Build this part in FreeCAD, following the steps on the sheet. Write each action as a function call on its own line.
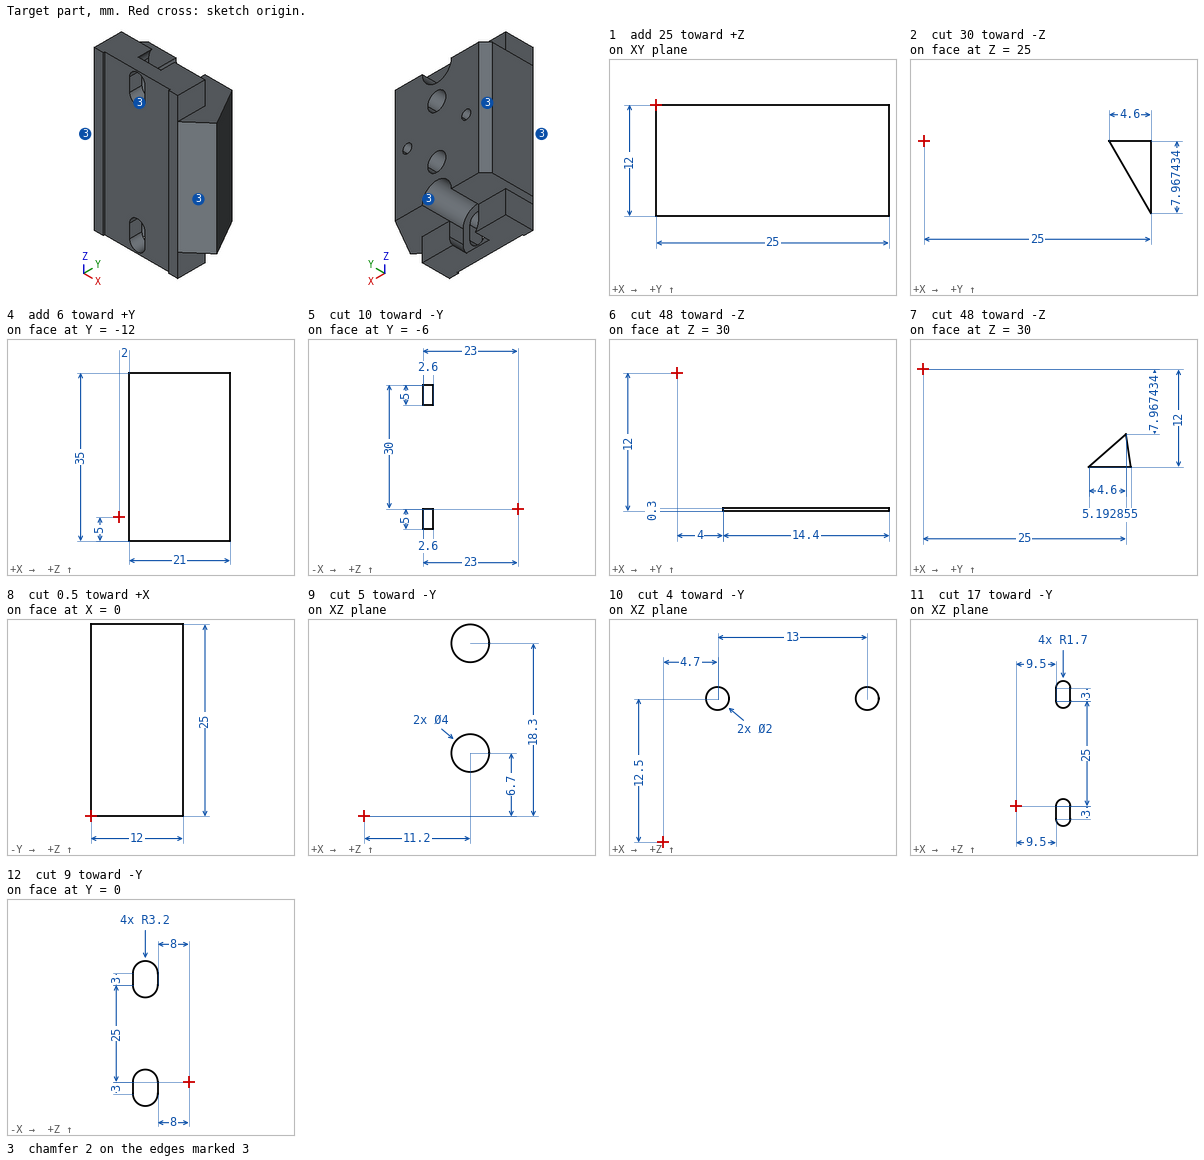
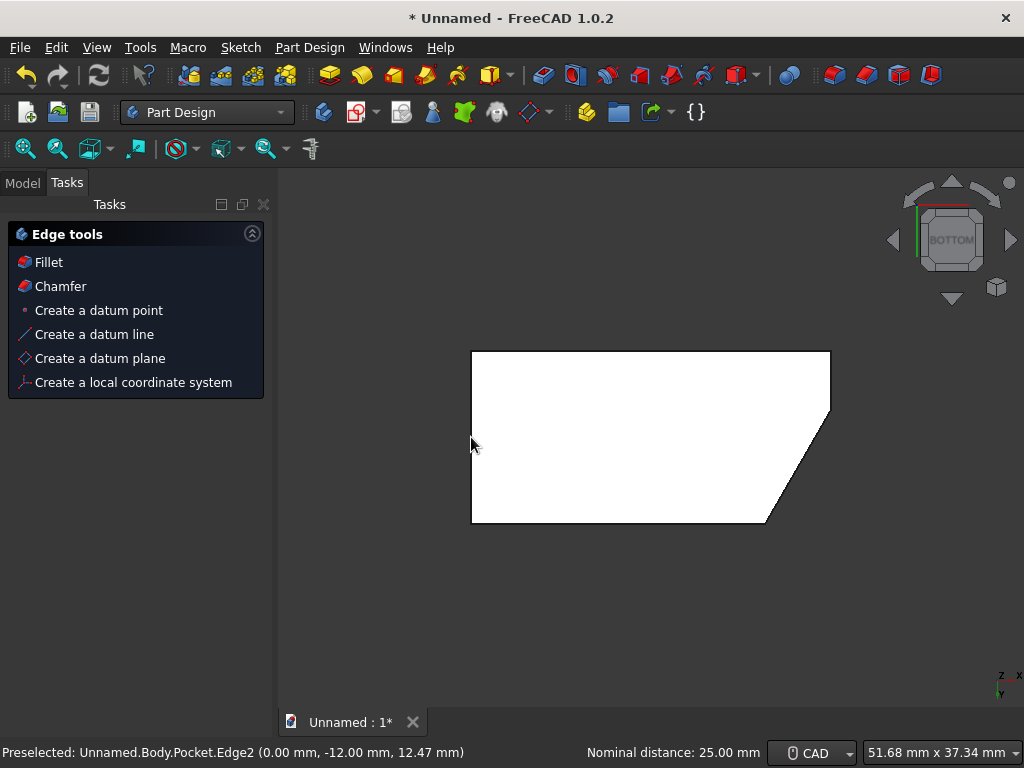
key(4)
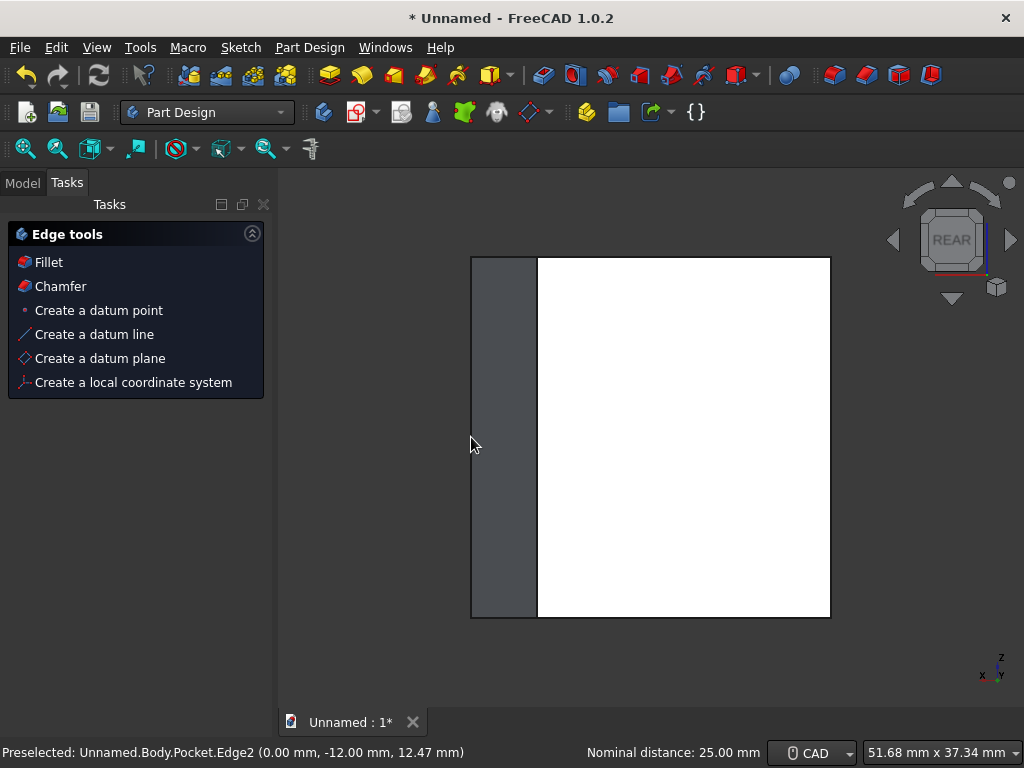
click(831, 437, ctrl)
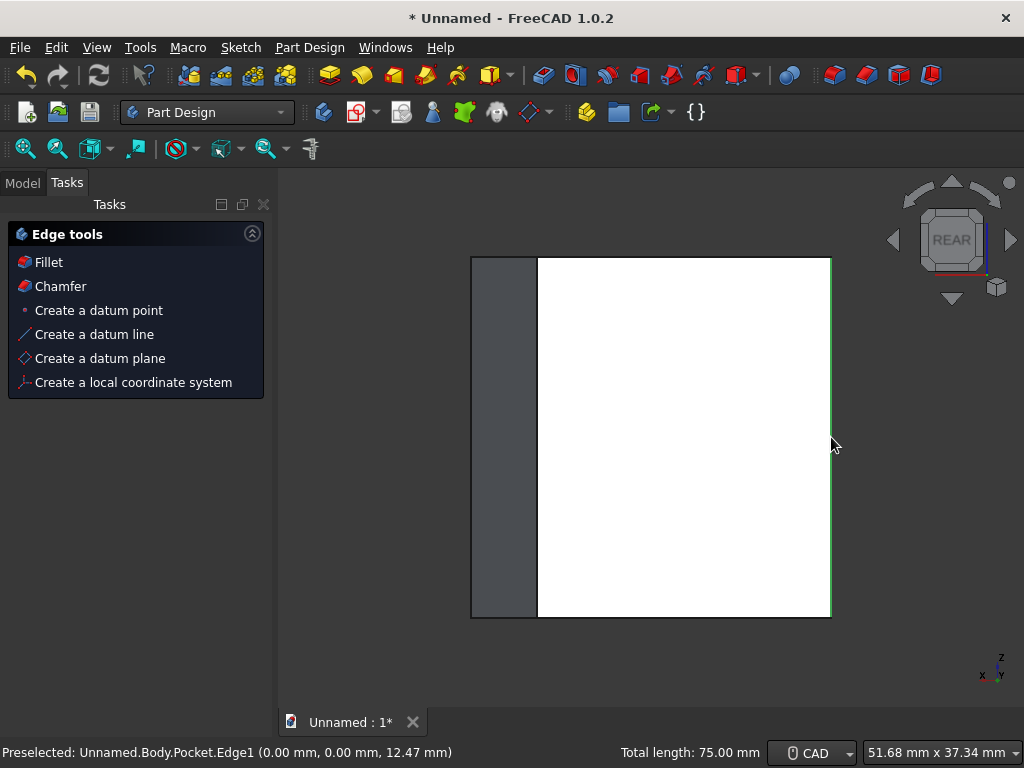
click(868, 76)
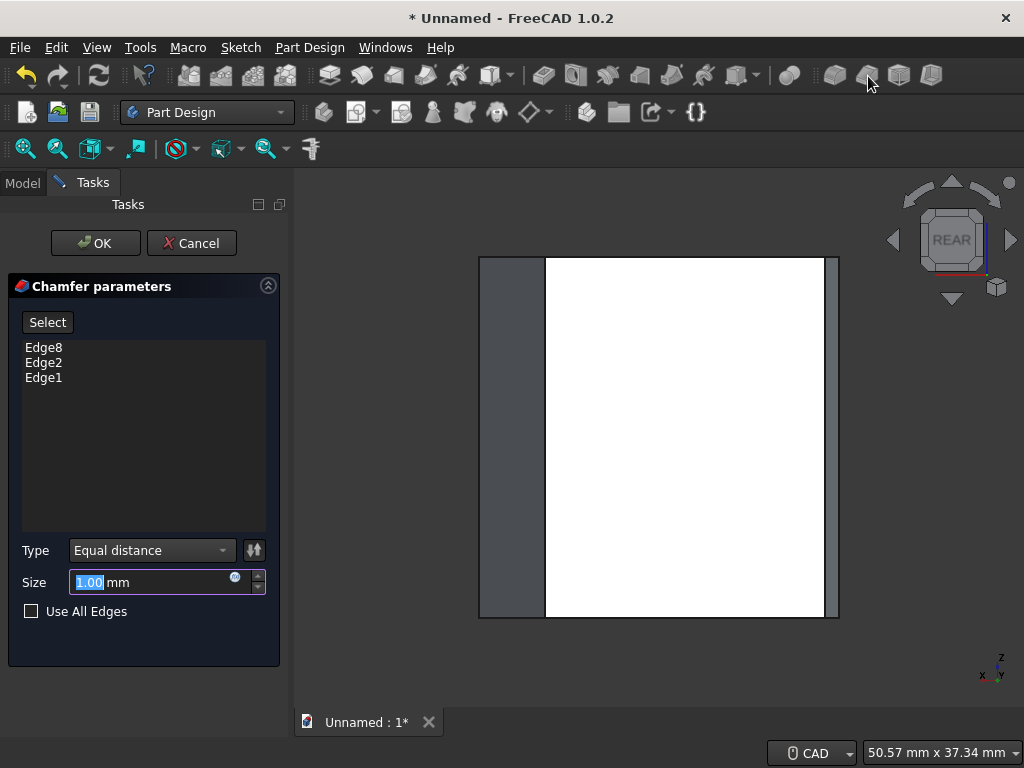
text(2)
key(Tab)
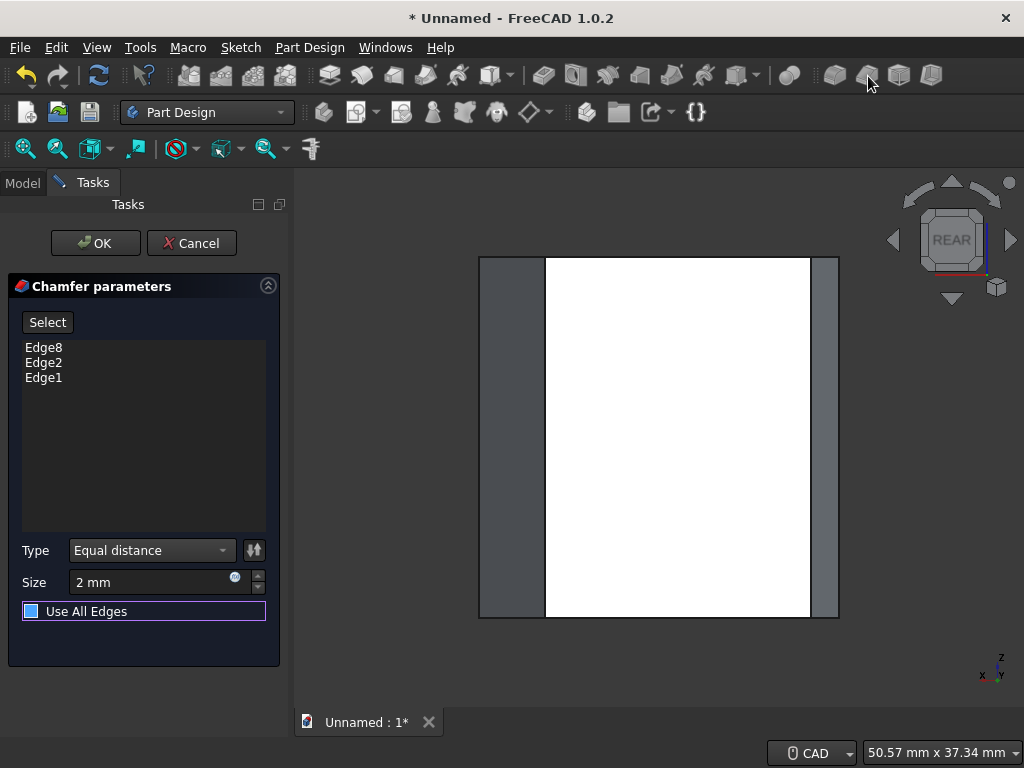
click(96, 243)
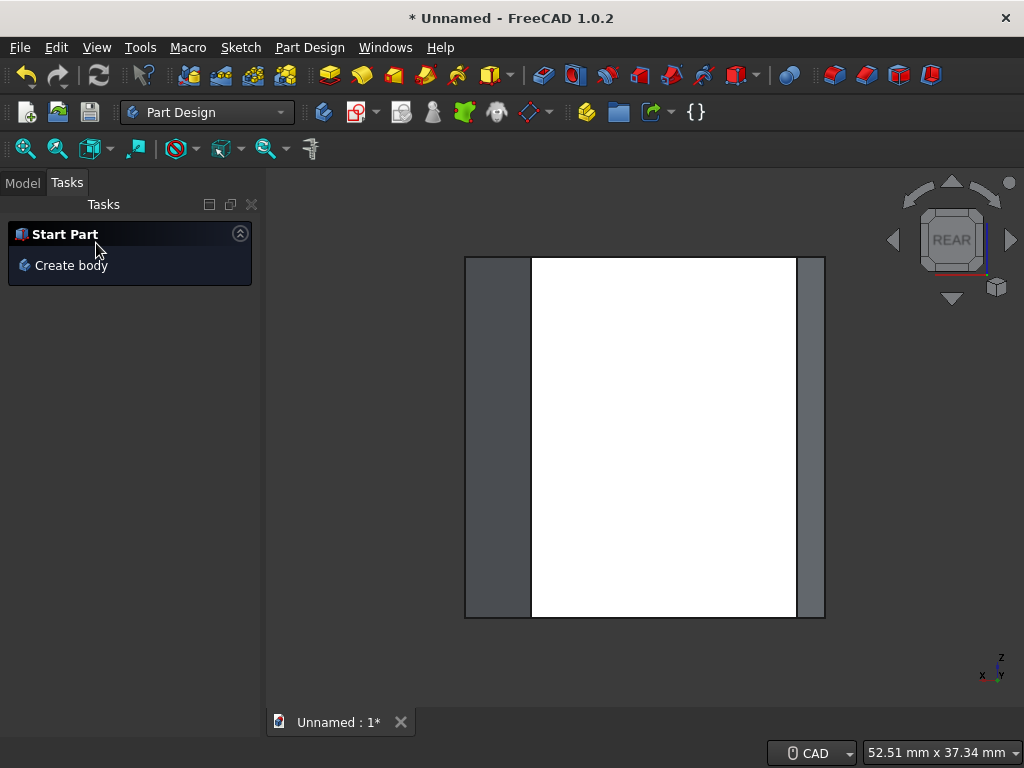
key(0)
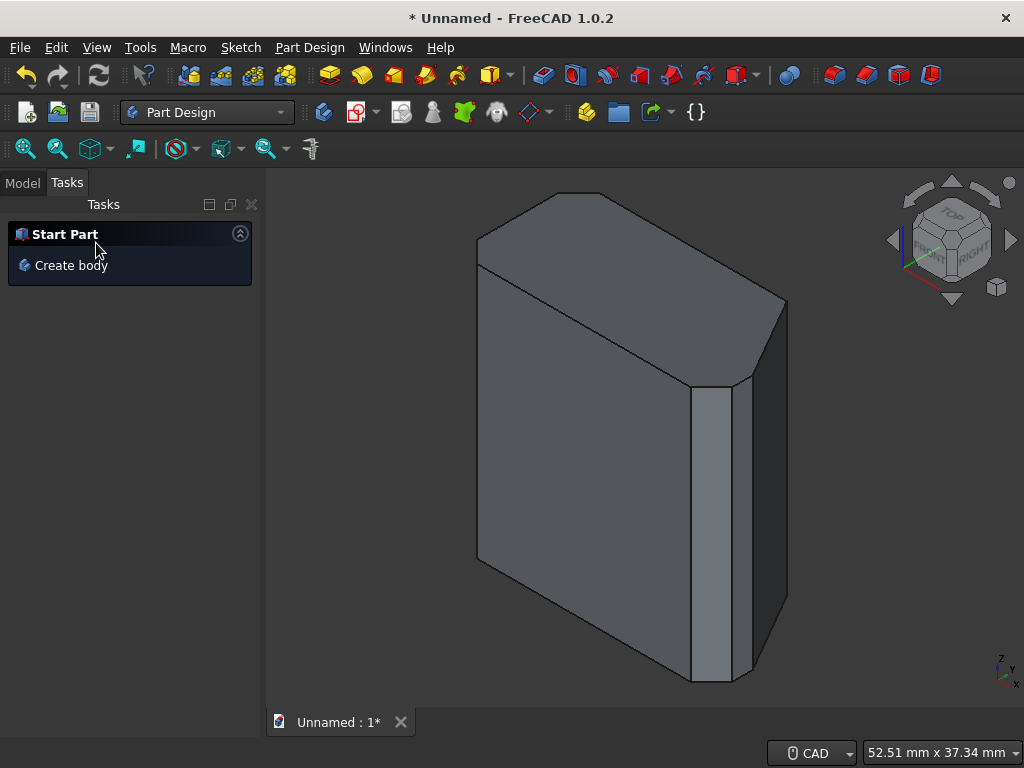
click(584, 472)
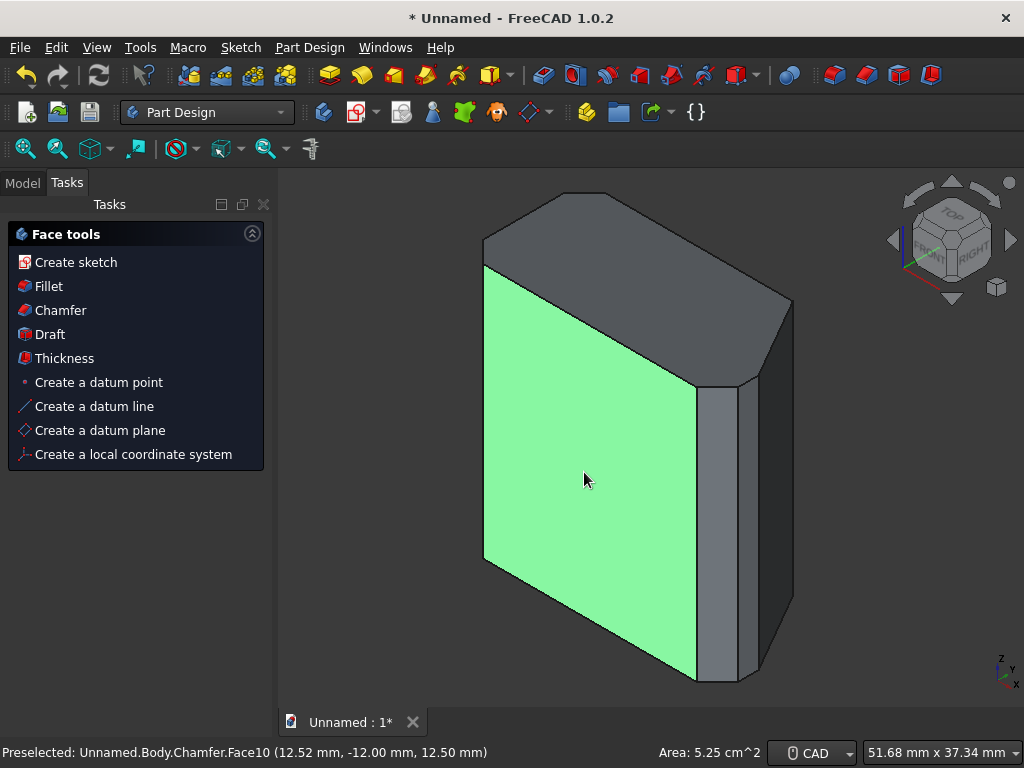
click(356, 112)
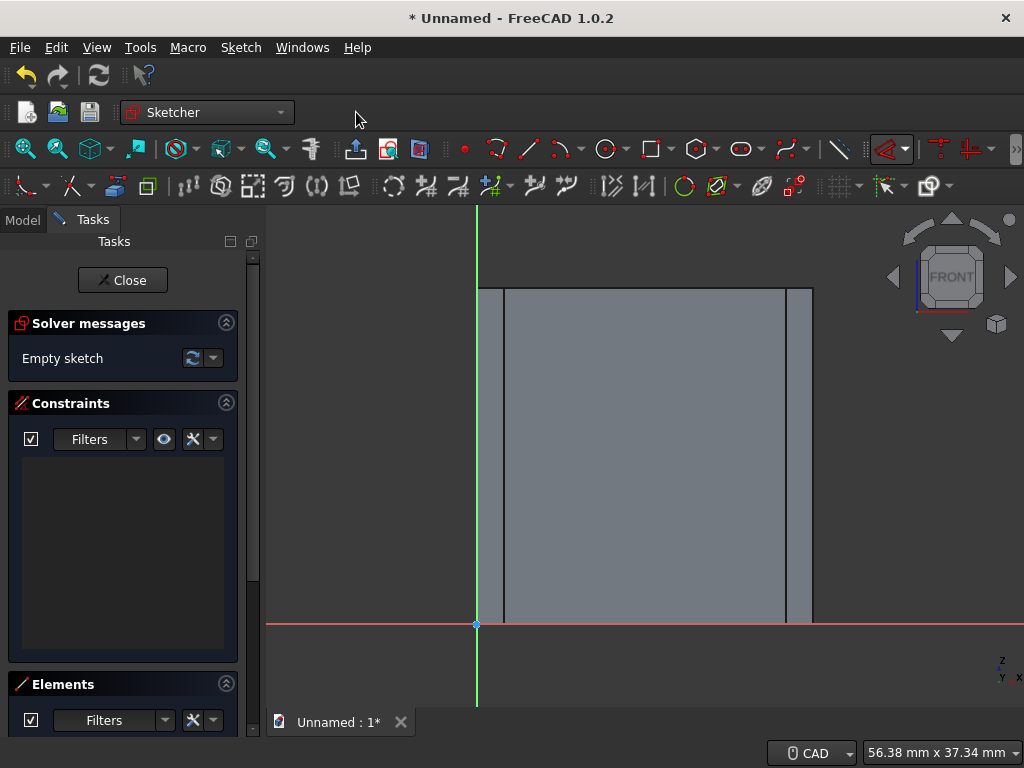
scroll(465, 456, down, 2)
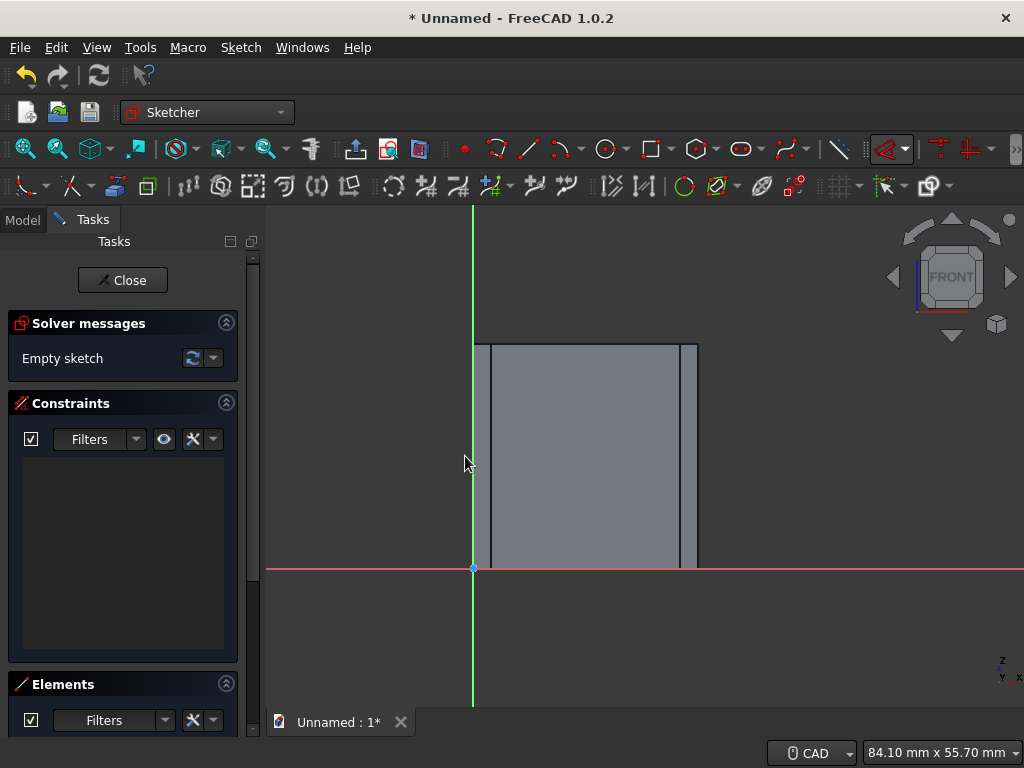
click(652, 150)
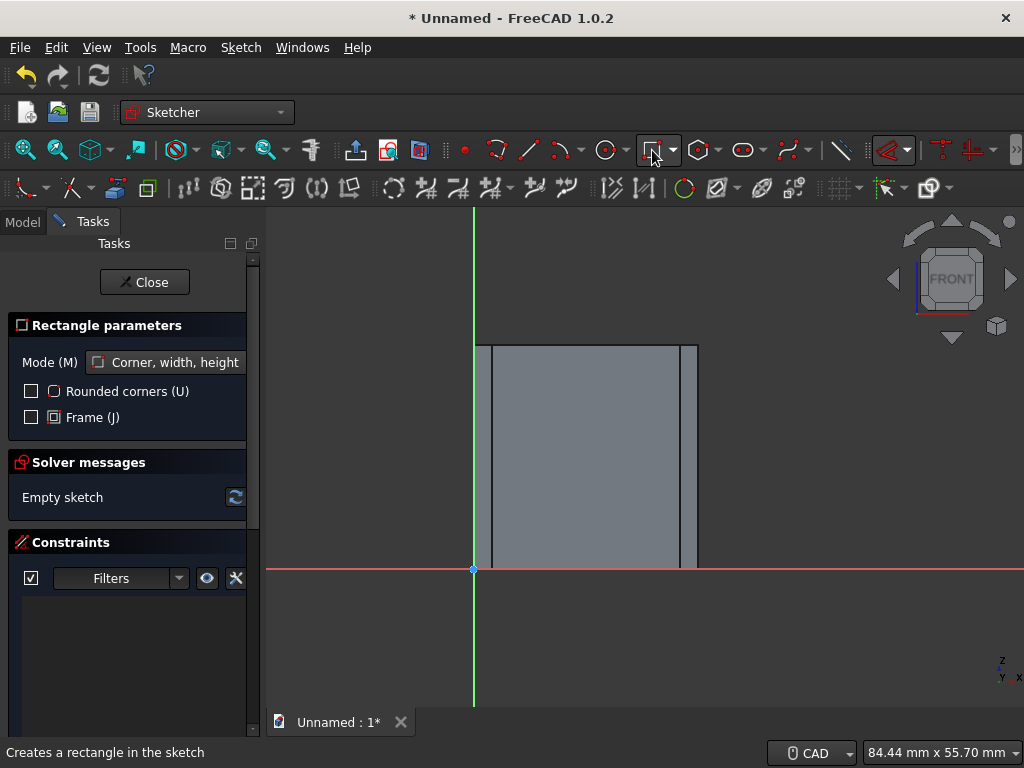
click(492, 300)
click(680, 614)
key(Escape)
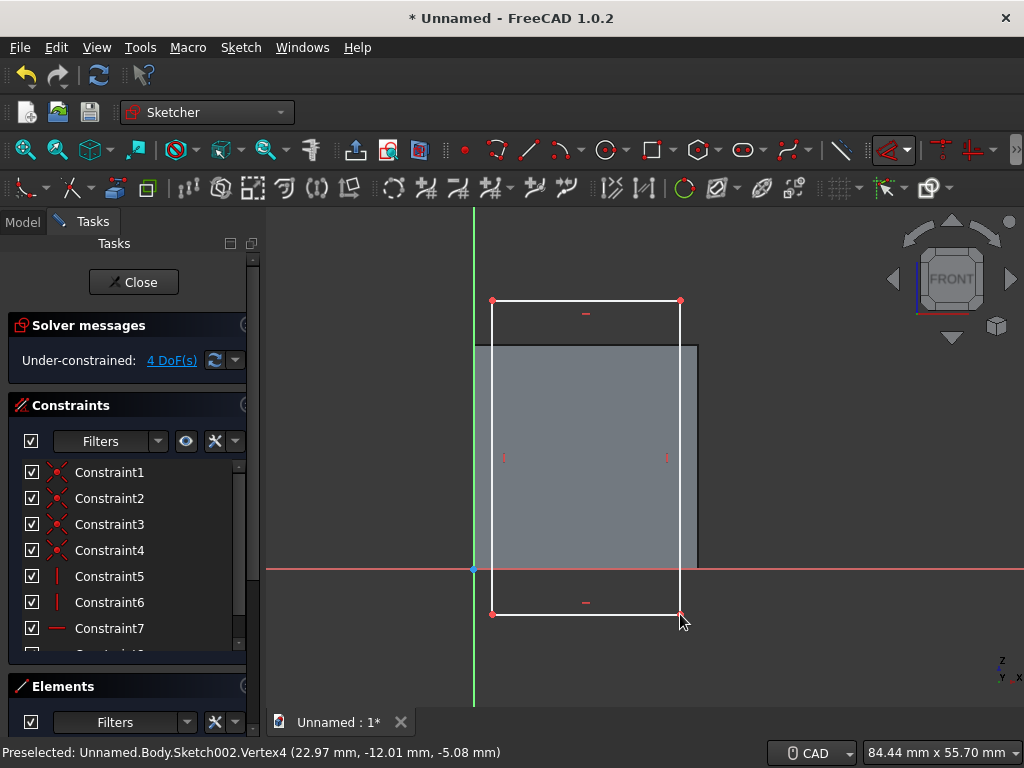
click(492, 395)